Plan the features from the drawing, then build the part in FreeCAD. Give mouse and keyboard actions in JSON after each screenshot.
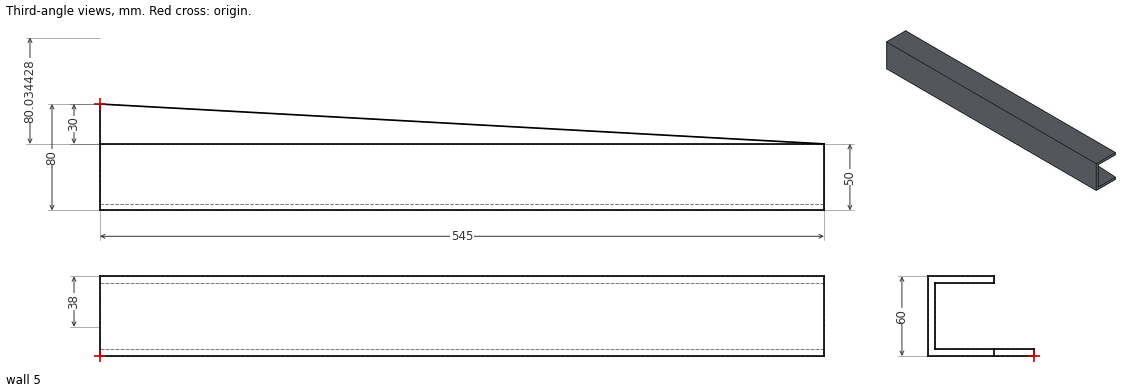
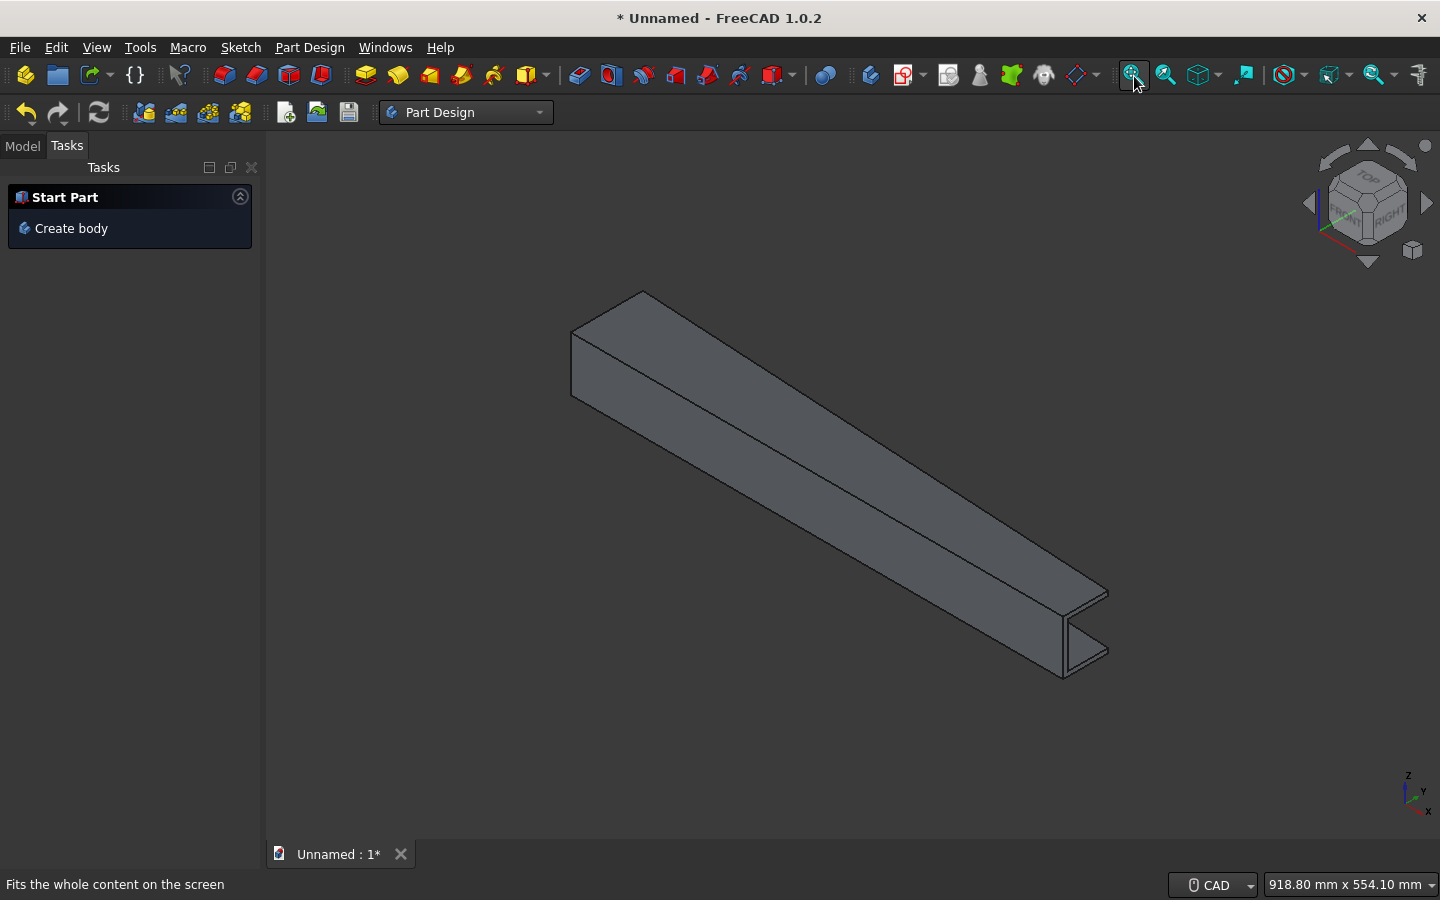
{"action": "left_click", "coordinate": [642, 331]}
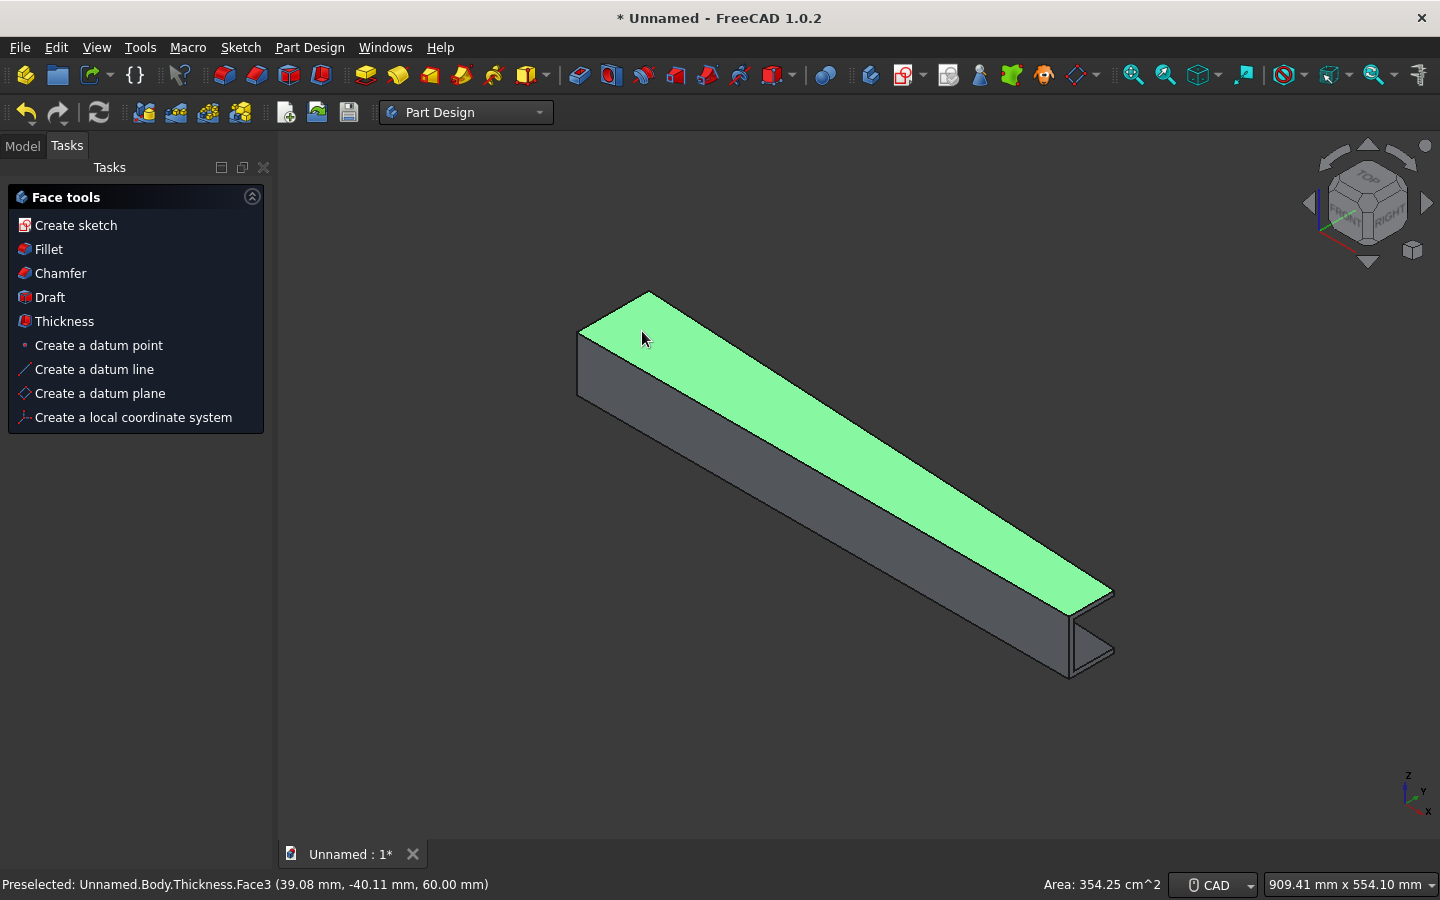
{"action": "left_click", "coordinate": [904, 76]}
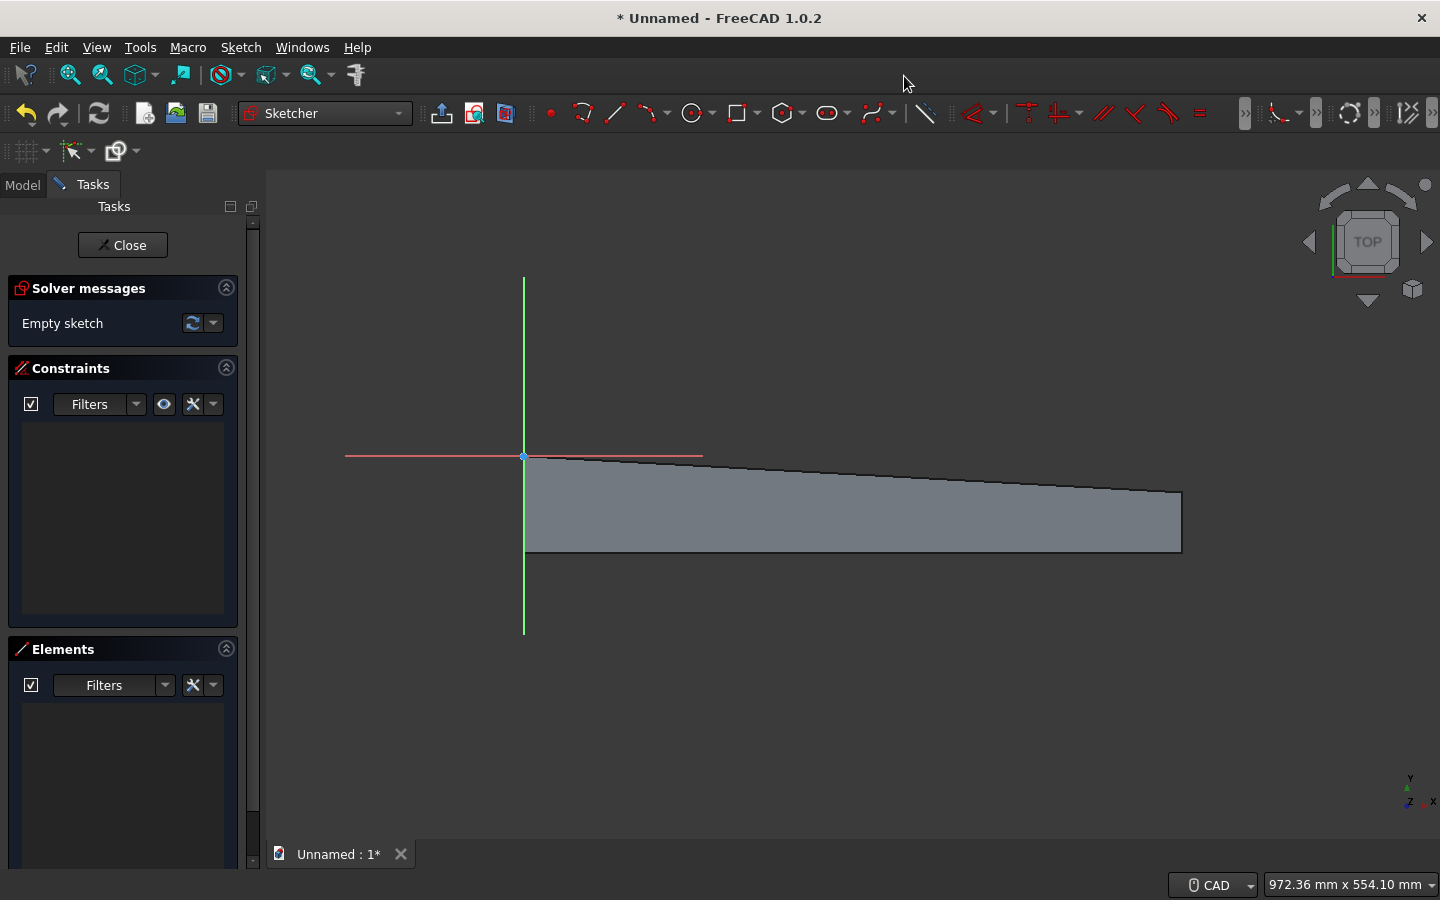
{"action": "key", "text": "g m"}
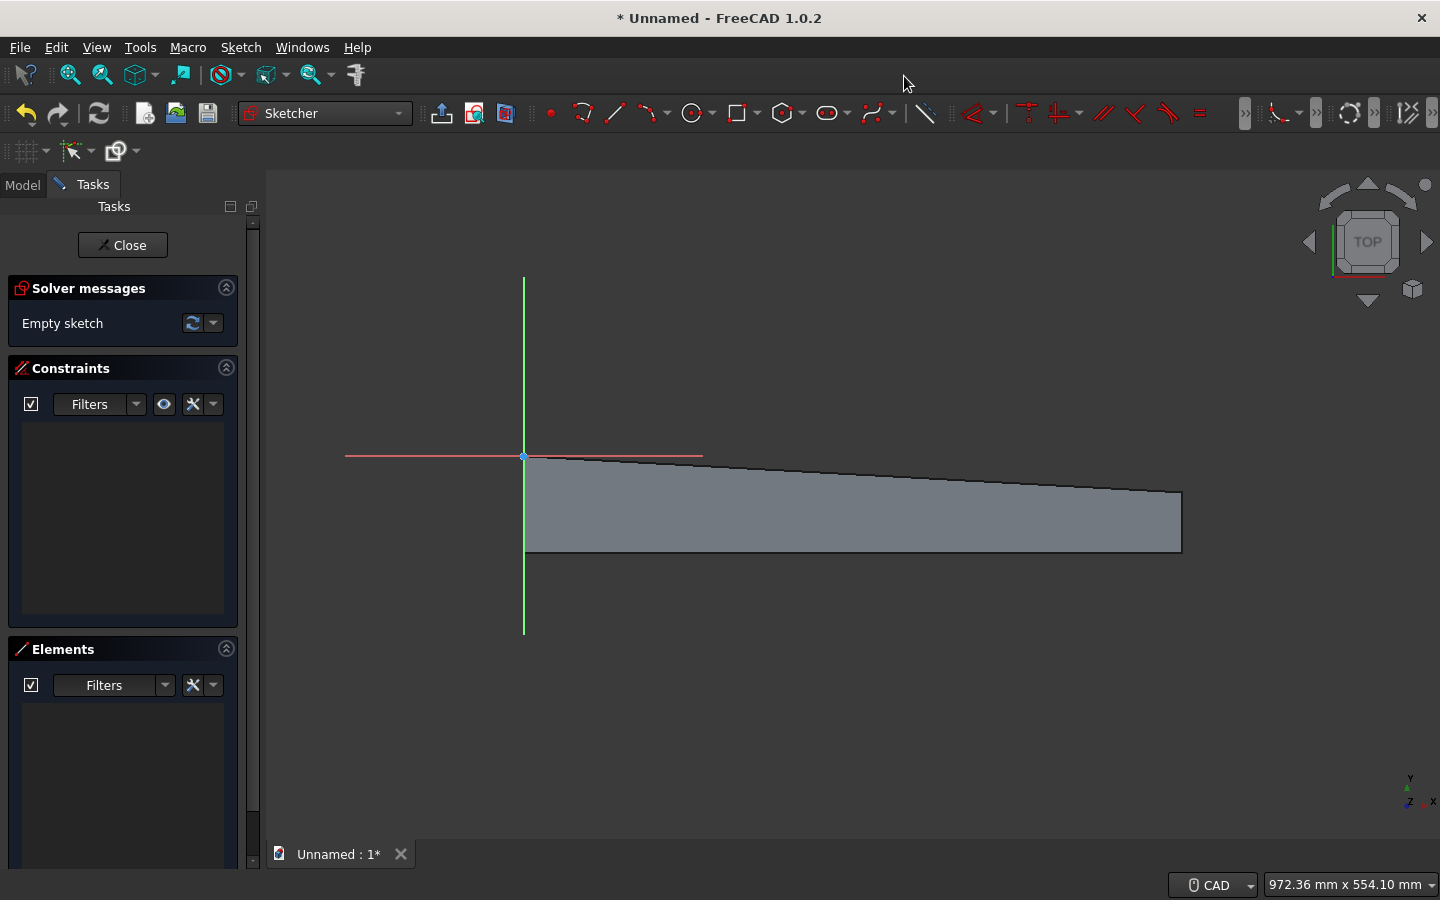
{"action": "left_click", "coordinate": [524, 492]}
{"action": "left_click", "coordinate": [1182, 492]}
{"action": "left_click", "coordinate": [533, 396]}
{"action": "left_click", "coordinate": [524, 493]}
{"action": "key", "text": "Escape"}
{"action": "key", "text": "Escape"}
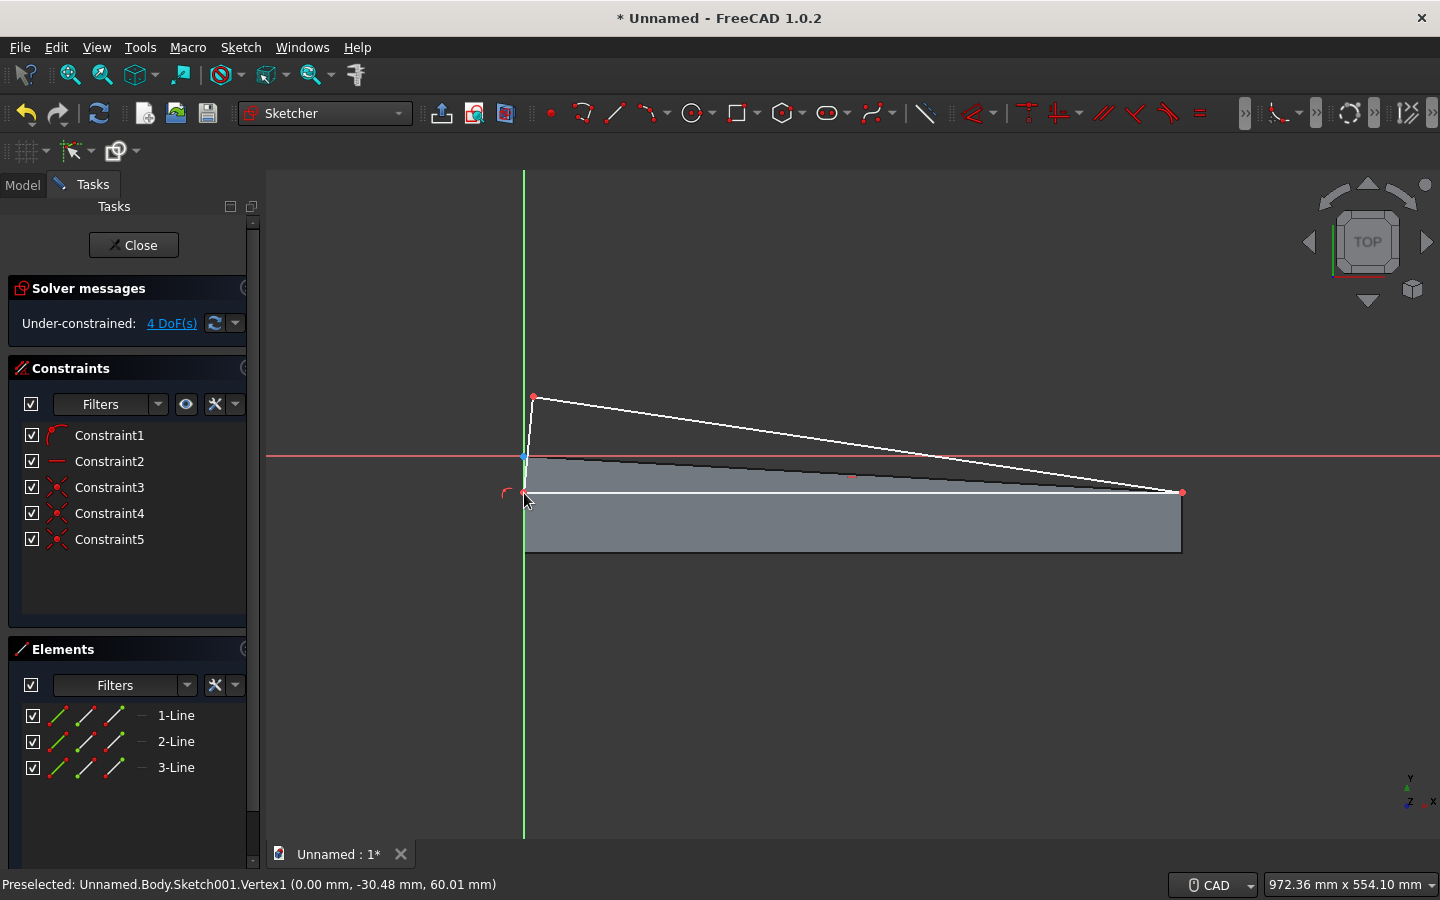
{"action": "left_click", "coordinate": [526, 474]}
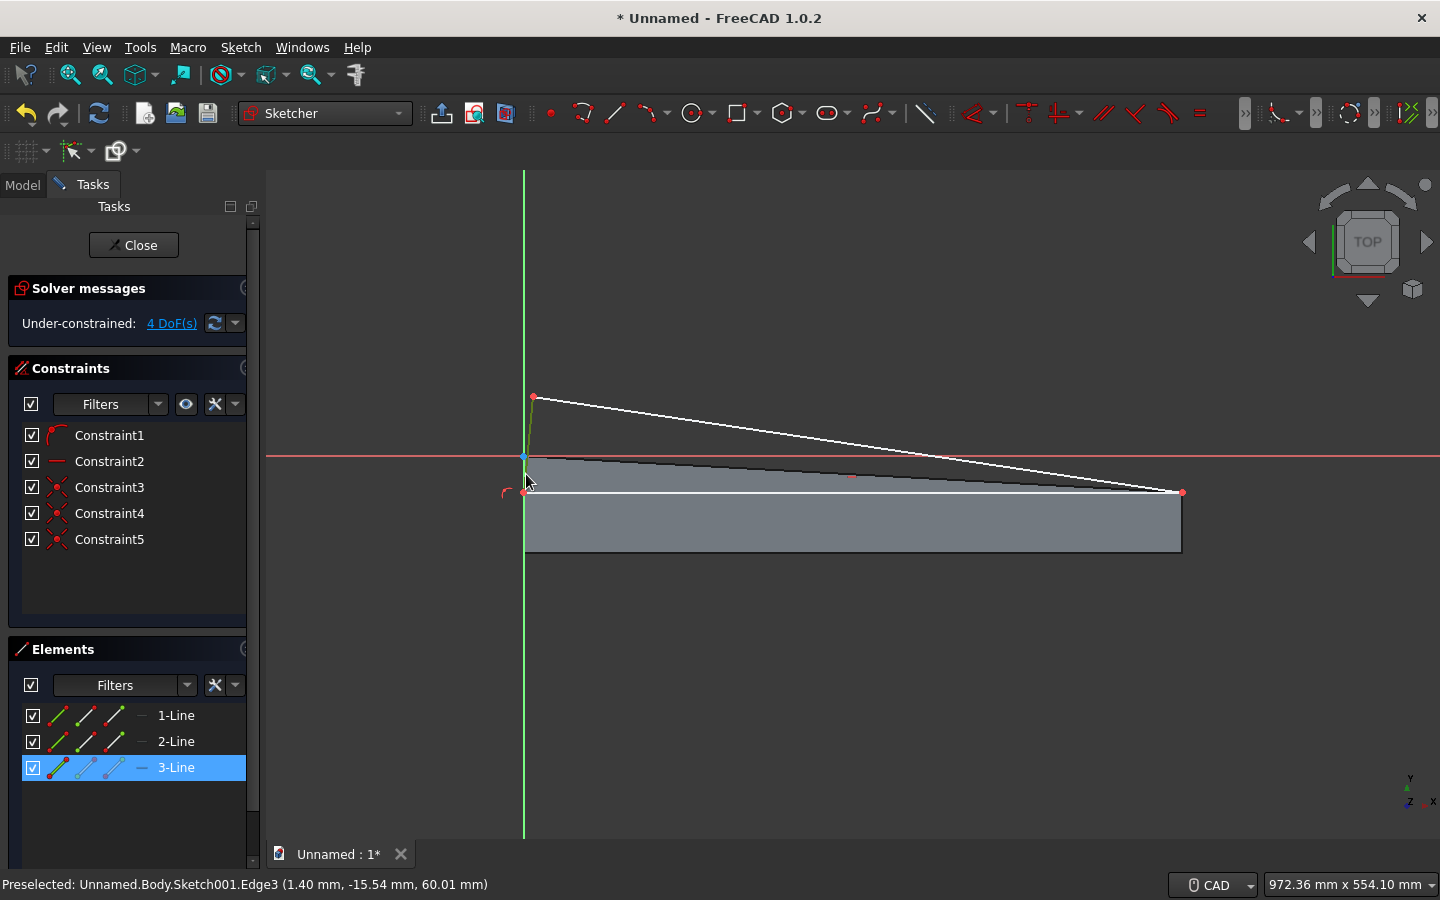
{"action": "key", "text": "v"}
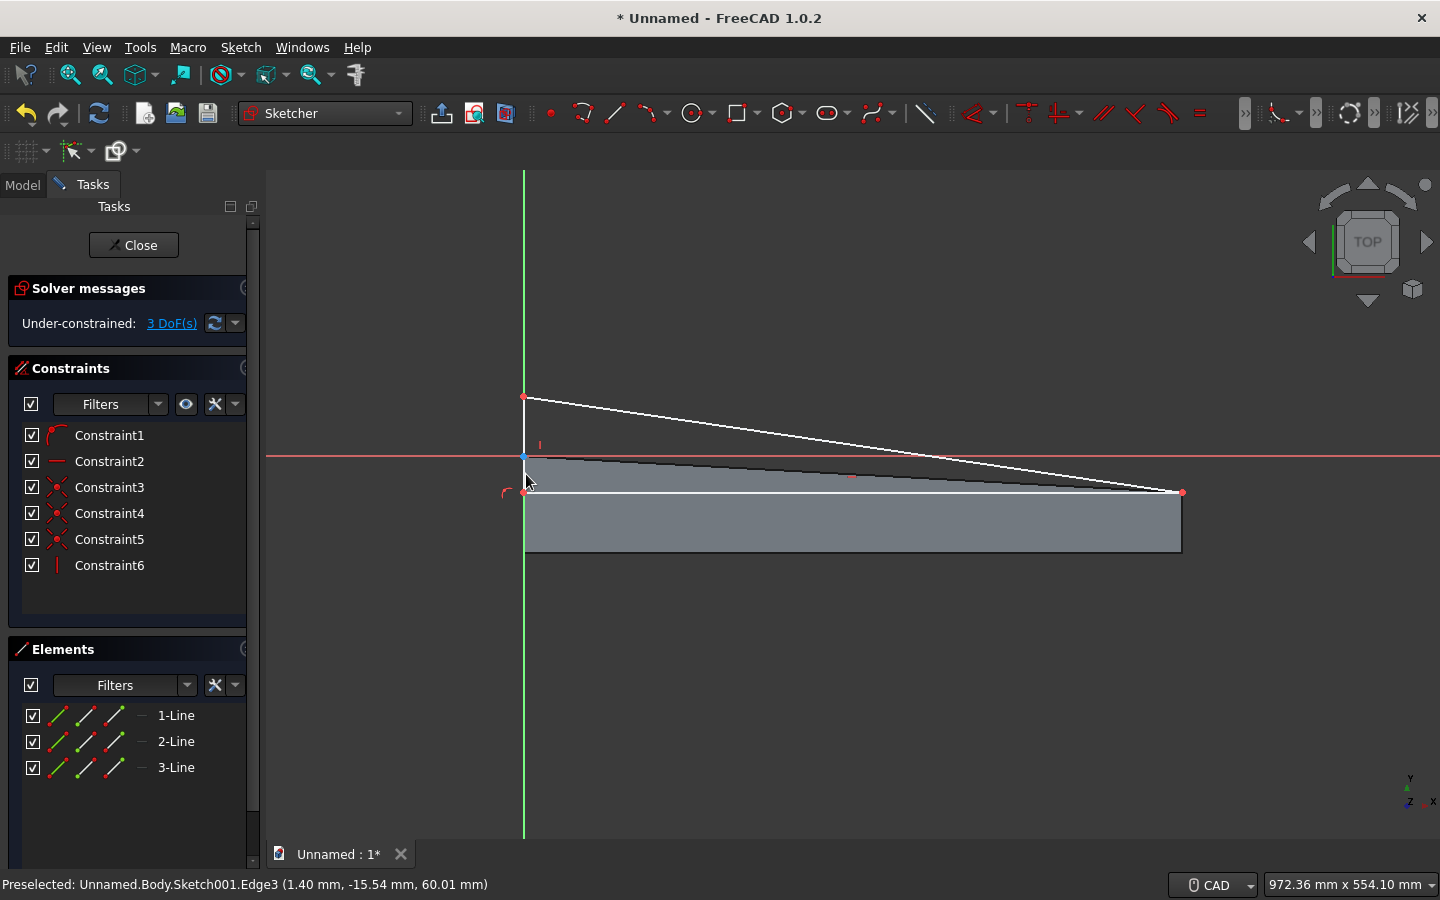
{"action": "key", "text": "d"}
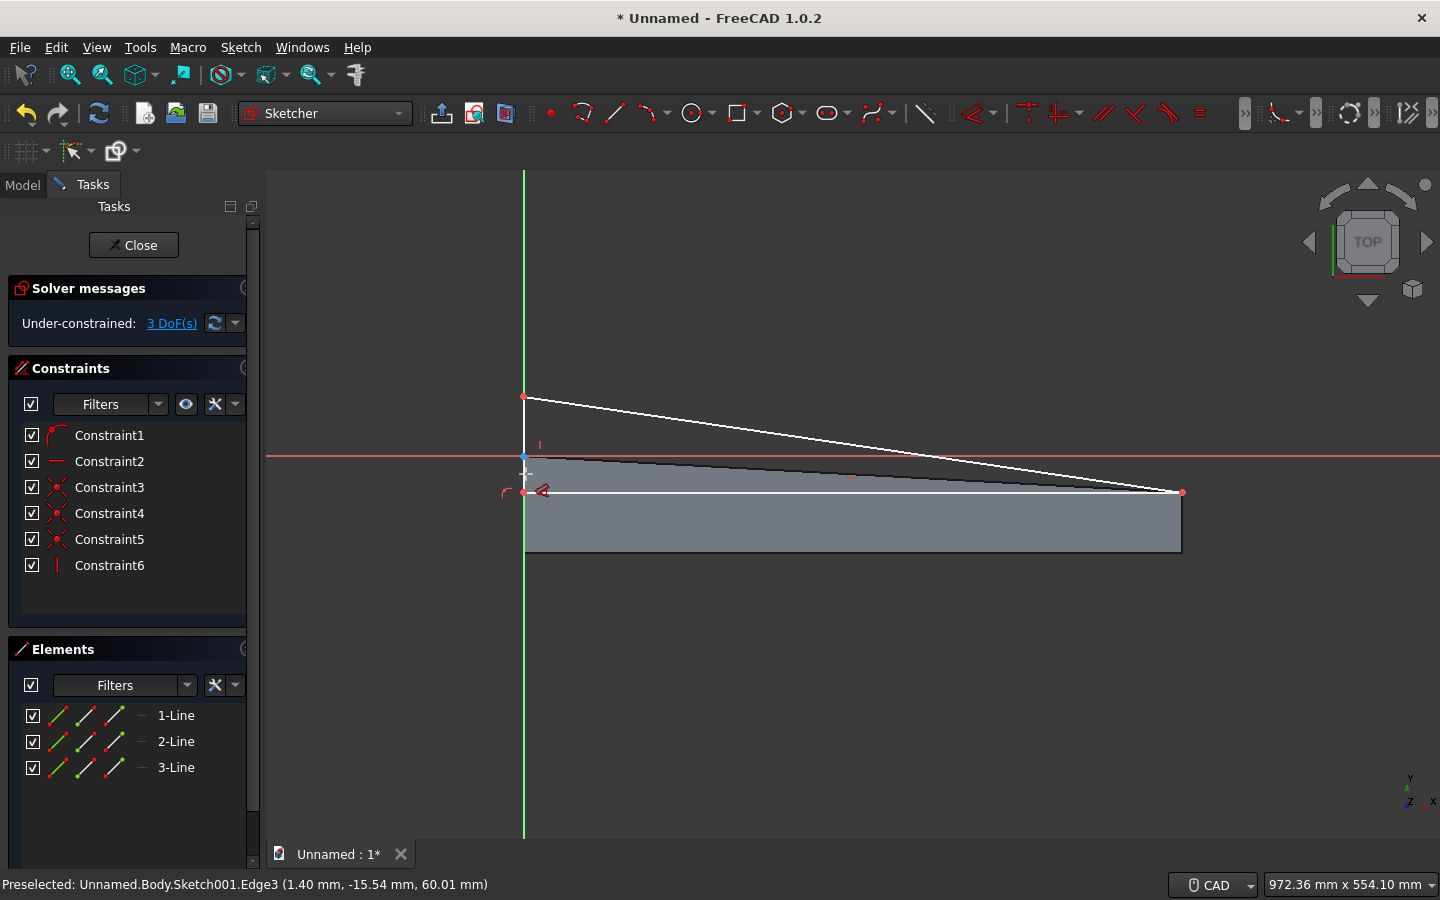
{"action": "left_click", "coordinate": [721, 493]}
{"action": "left_click", "coordinate": [853, 527]}